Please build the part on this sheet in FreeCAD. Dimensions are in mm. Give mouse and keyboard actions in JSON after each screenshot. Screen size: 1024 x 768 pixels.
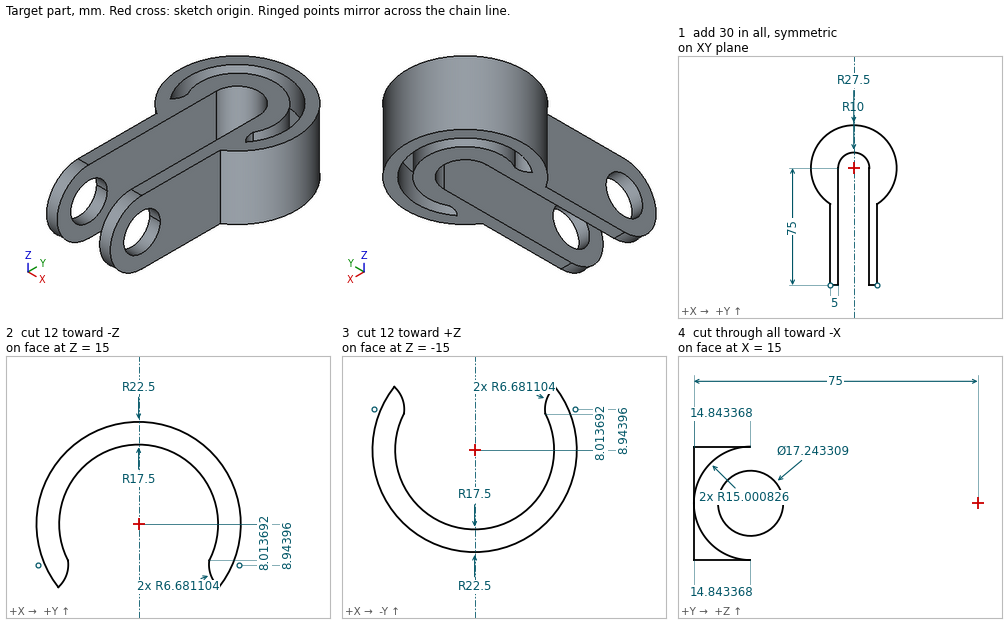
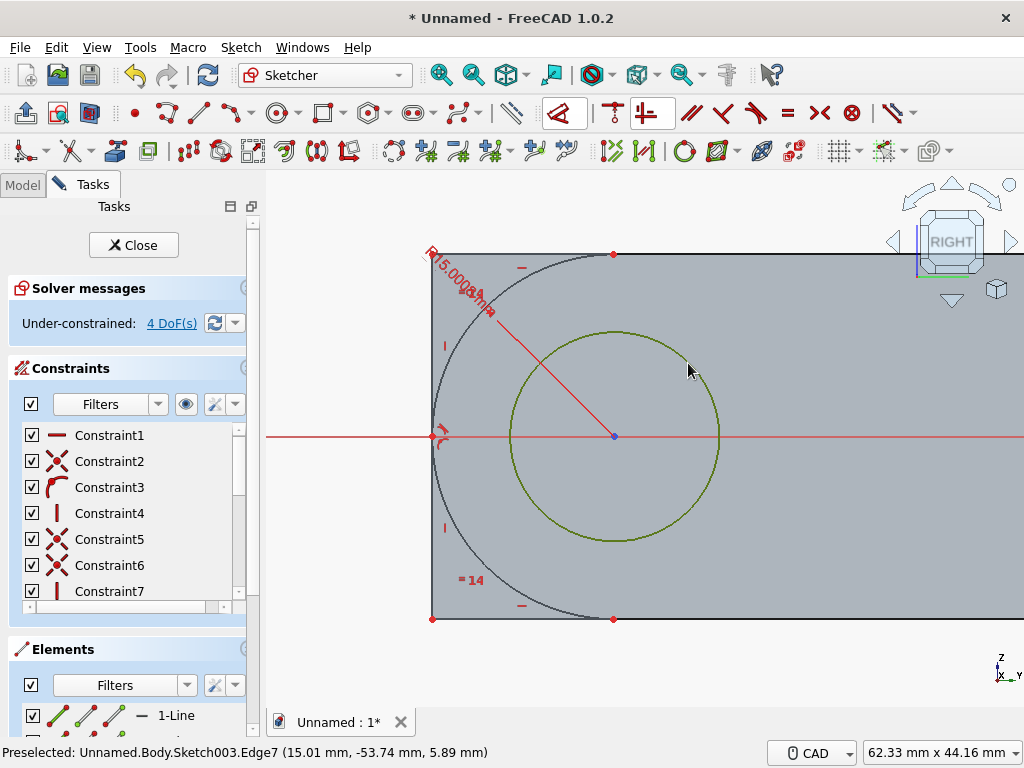
{"action": "key", "text": "k o"}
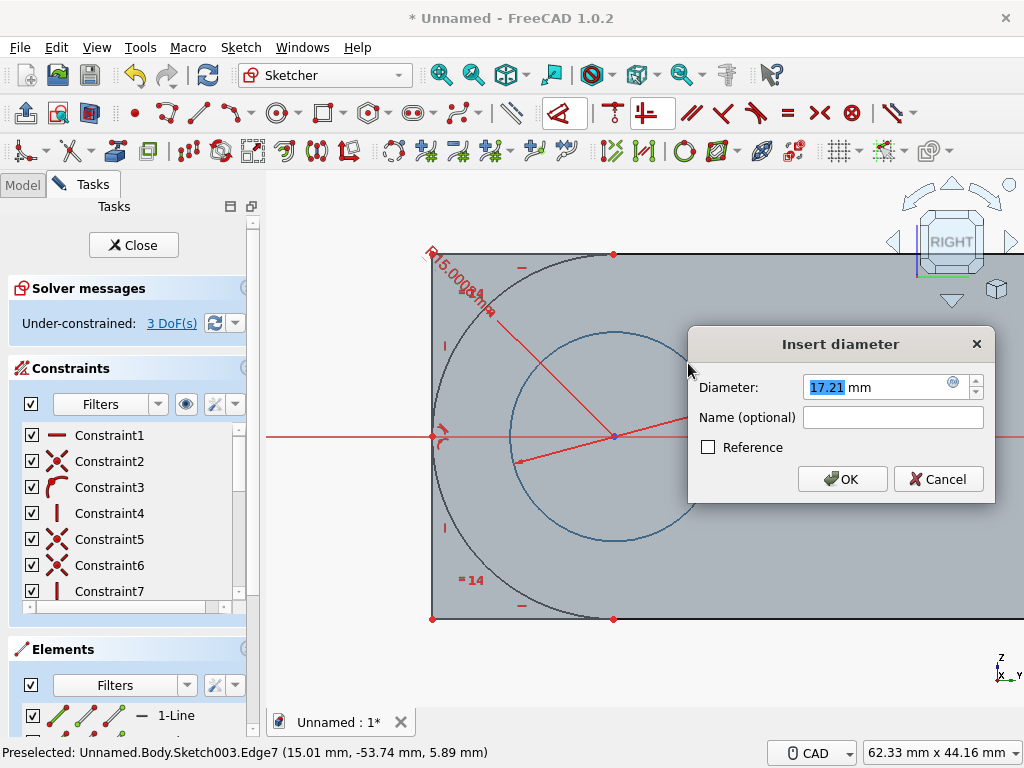
{"action": "type", "text": "17.243309"}
{"action": "key", "text": "Return"}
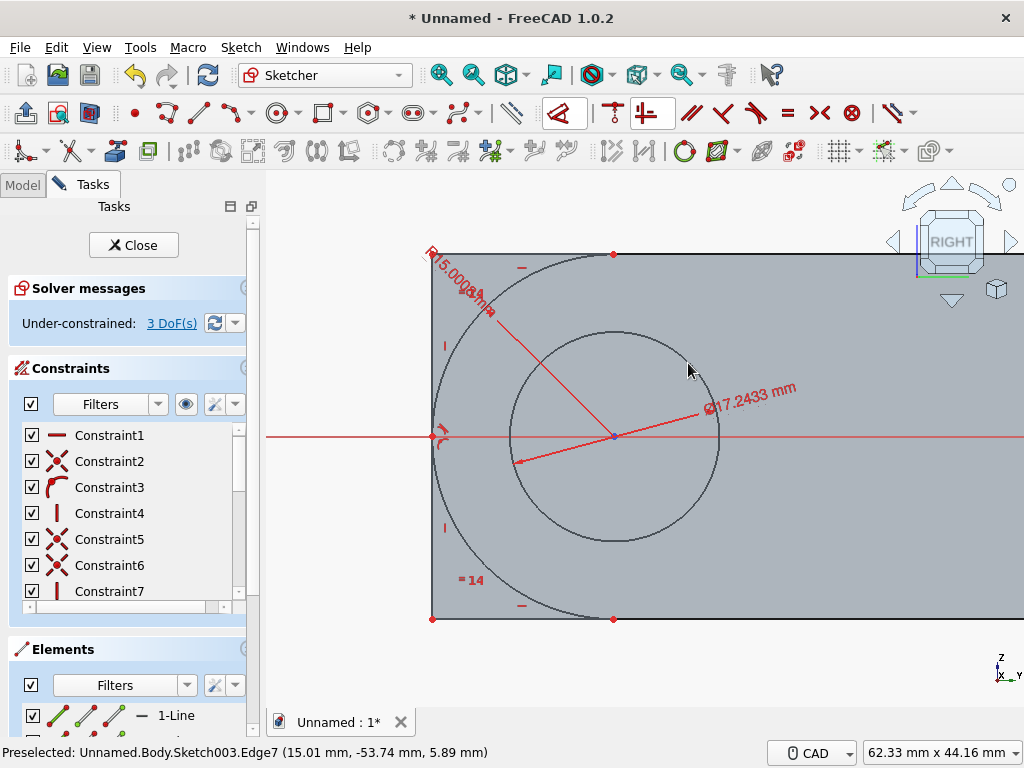
{"action": "left_click", "coordinate": [432, 254]}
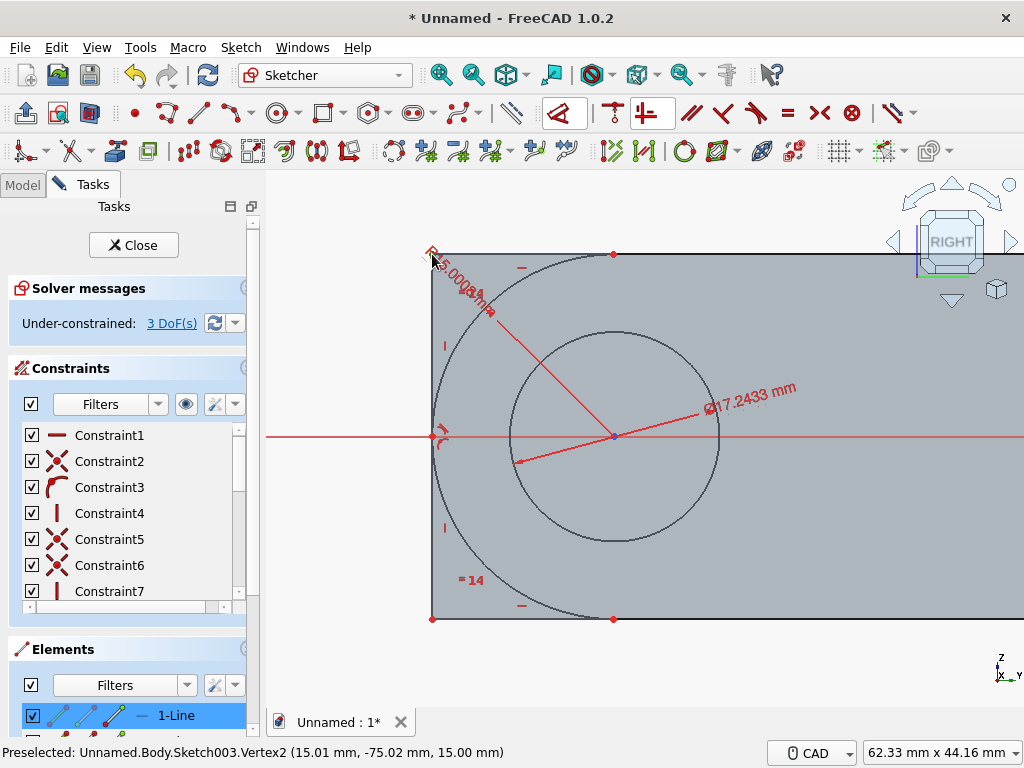
{"action": "key", "text": "l"}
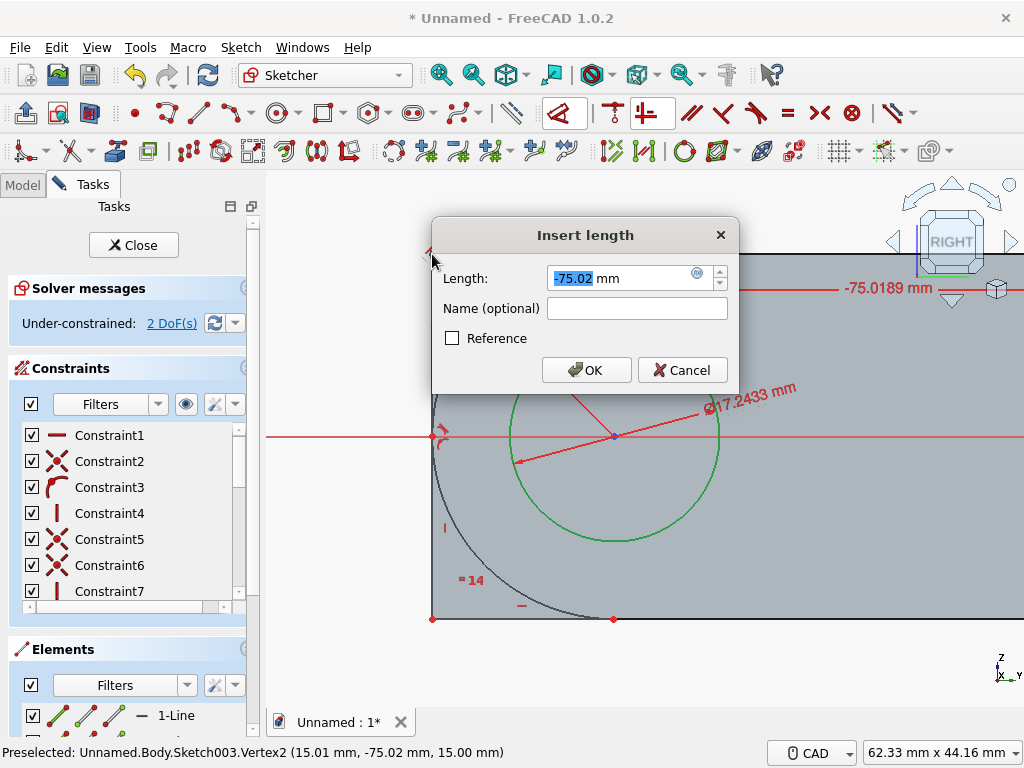
{"action": "type", "text": "-75"}
{"action": "key", "text": "Return"}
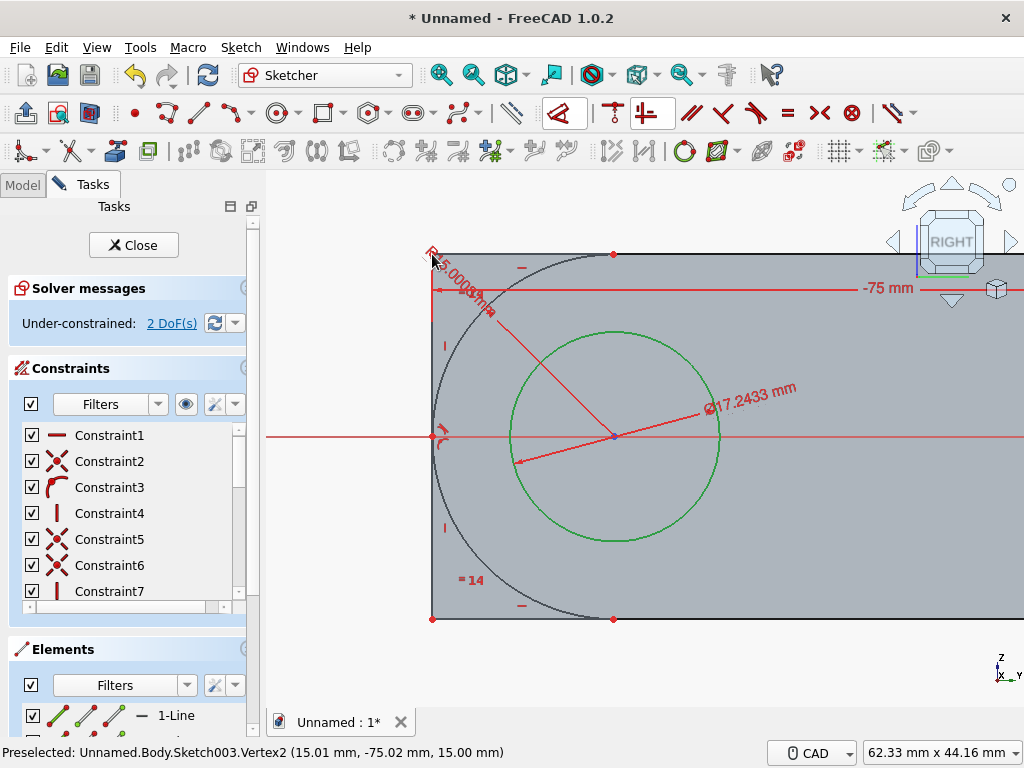
{"action": "left_click", "coordinate": [487, 254]}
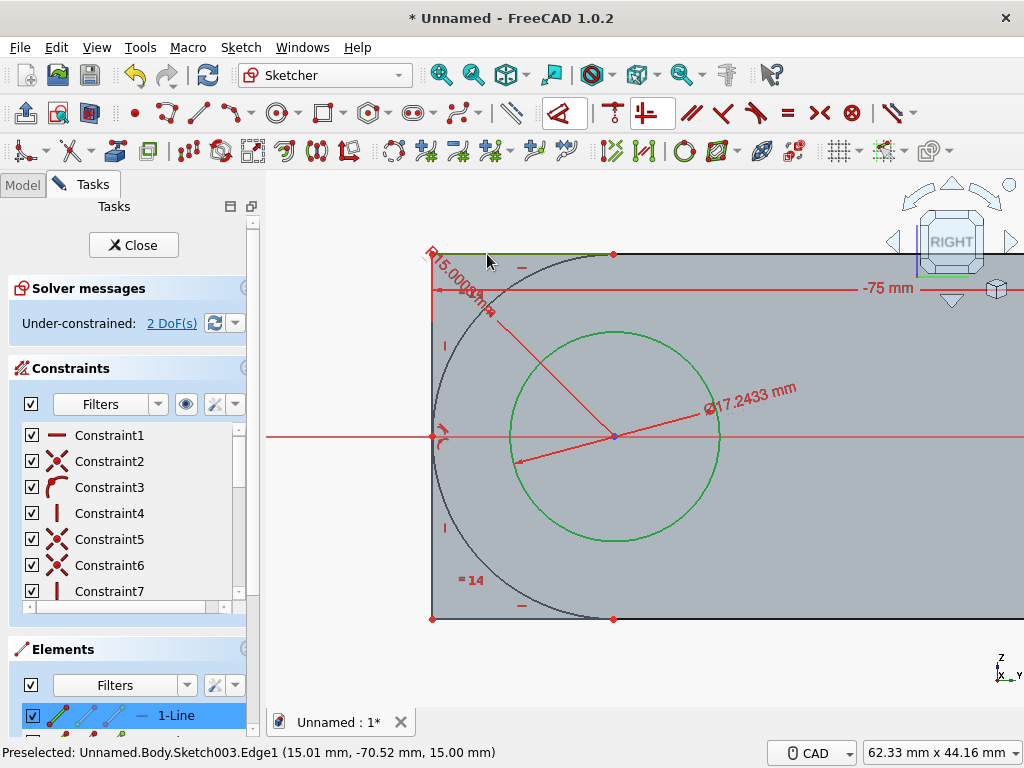
{"action": "key", "text": "l"}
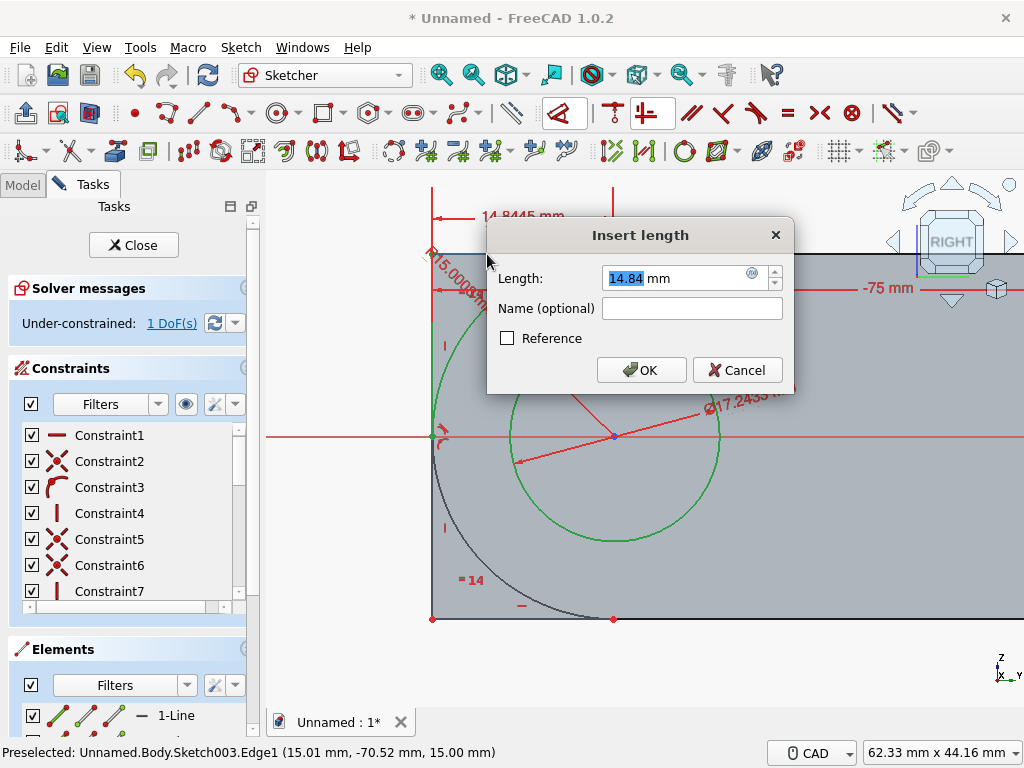
{"action": "type", "text": "14.843368"}
{"action": "key", "text": "Return"}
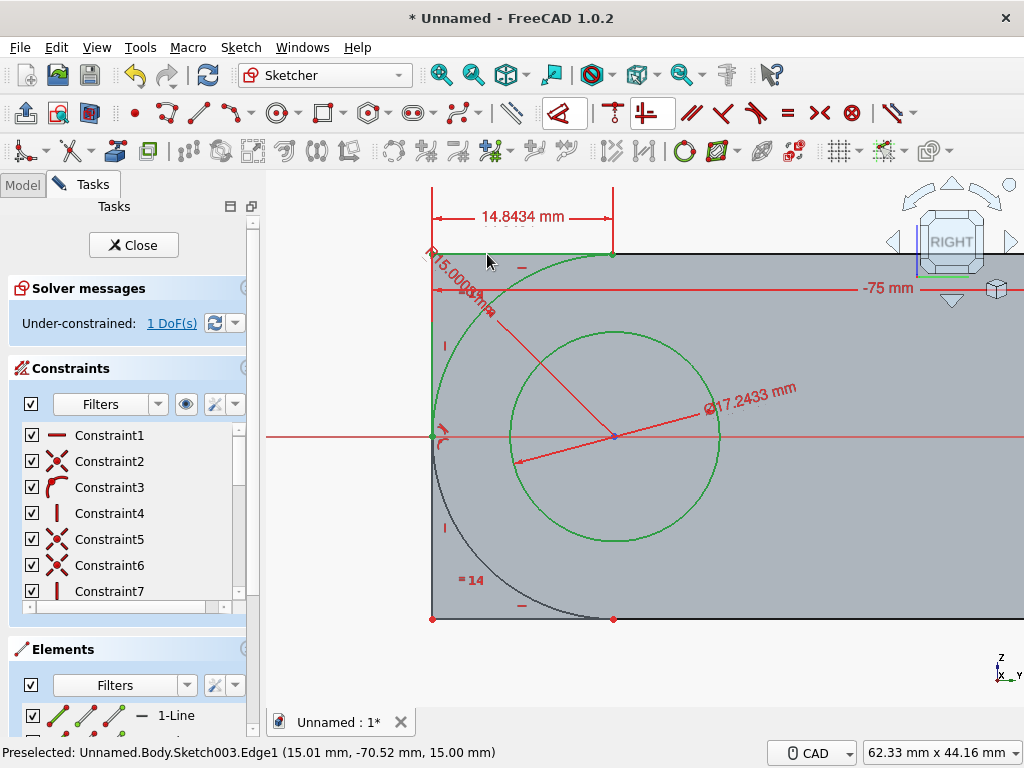
{"action": "left_click", "coordinate": [487, 619]}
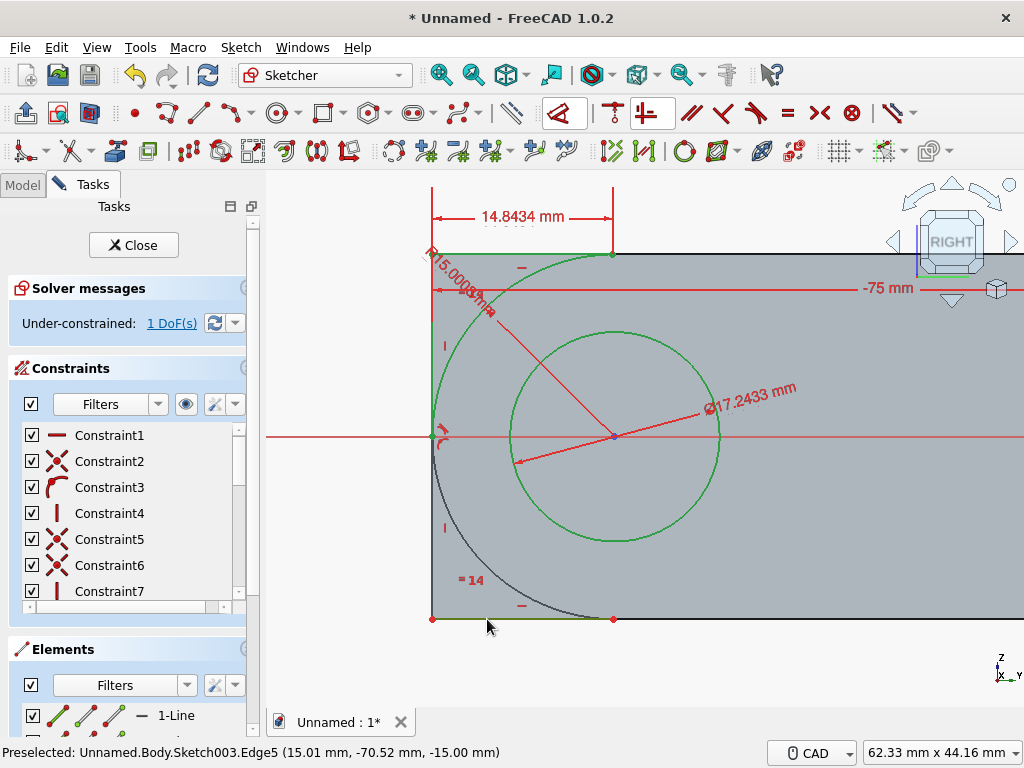
{"action": "key", "text": "l"}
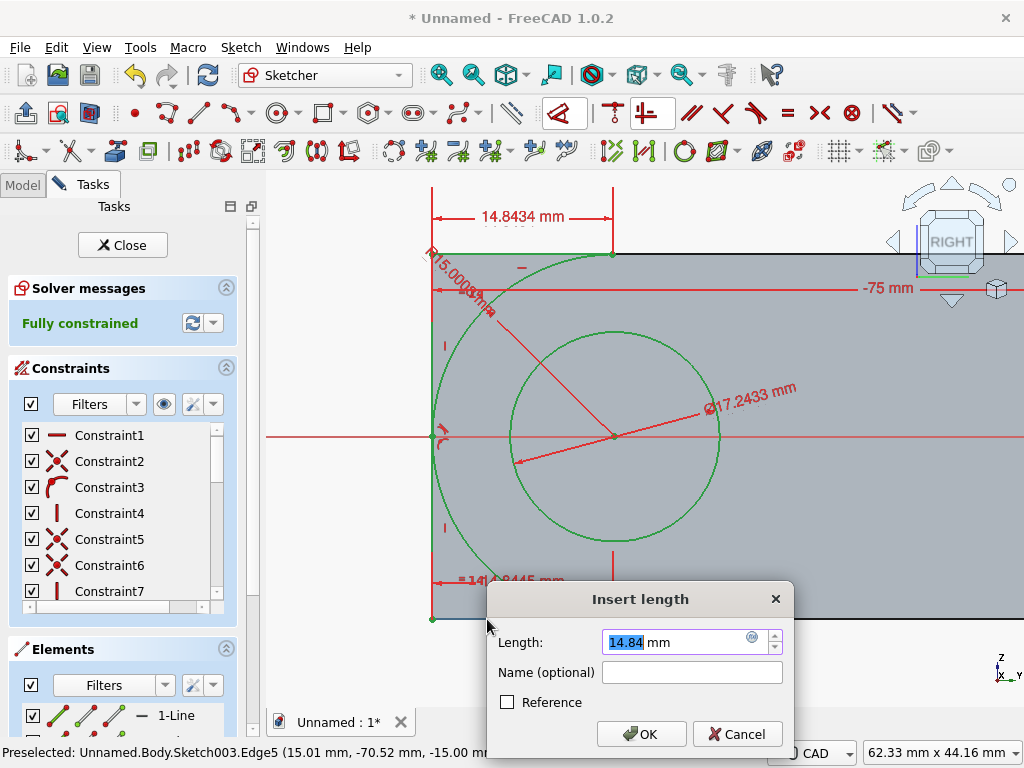
{"action": "type", "text": "14.843368"}
{"action": "key", "text": "Return"}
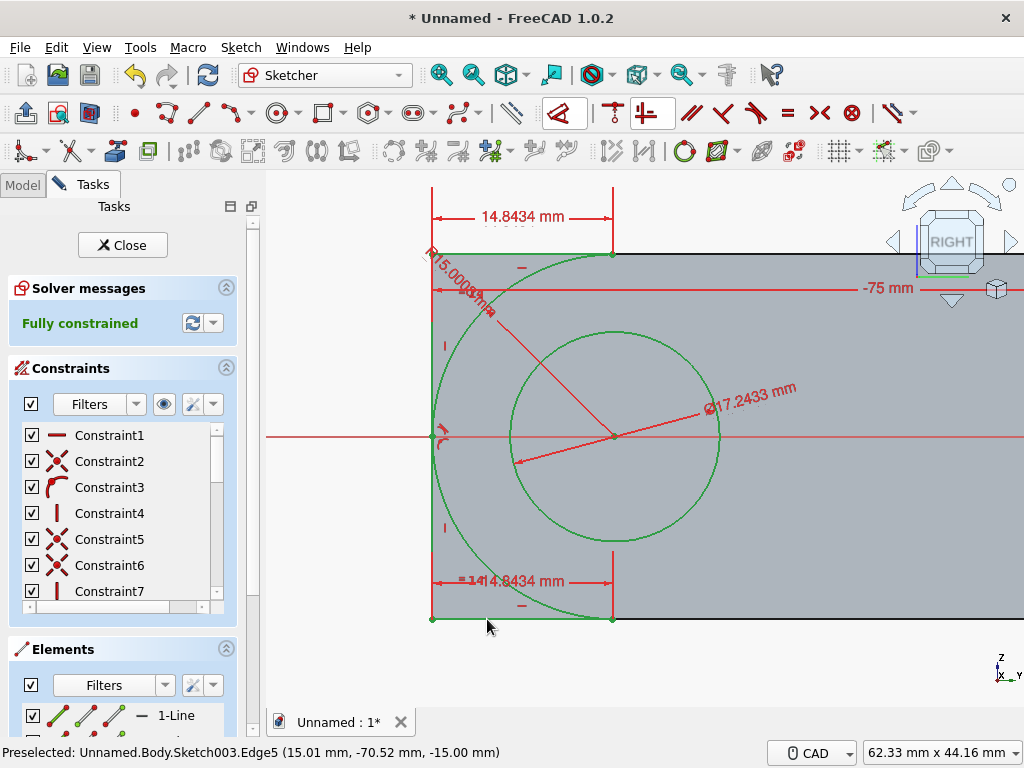
{"action": "left_click", "coordinate": [123, 245]}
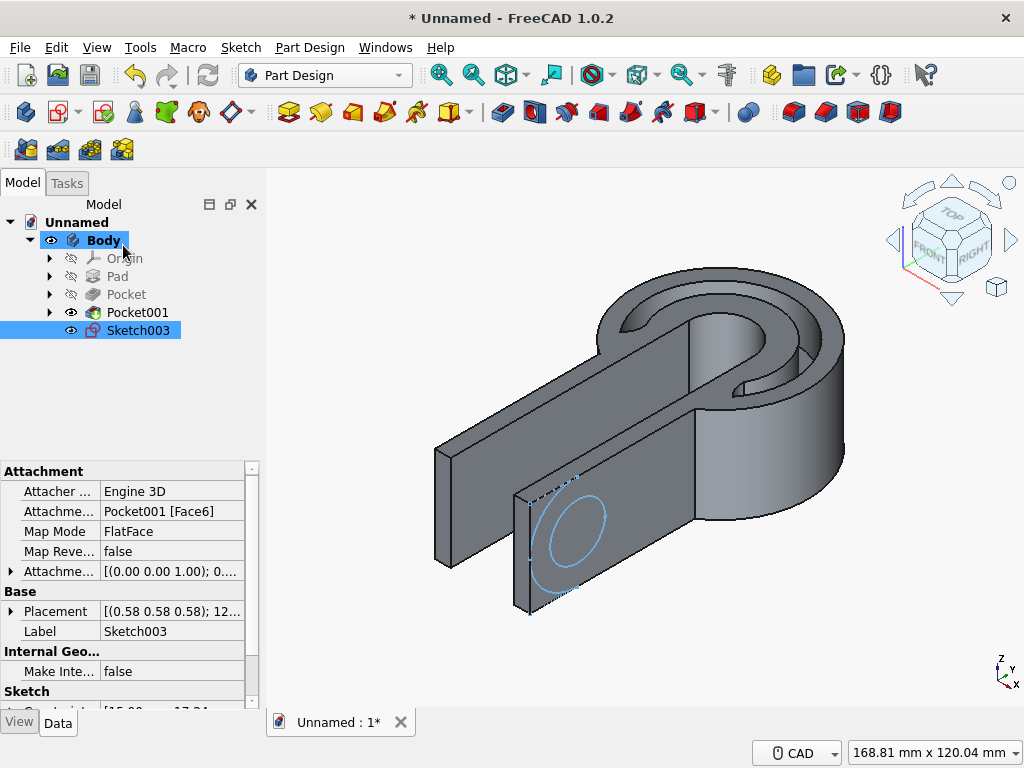
{"action": "left_click", "coordinate": [504, 112]}